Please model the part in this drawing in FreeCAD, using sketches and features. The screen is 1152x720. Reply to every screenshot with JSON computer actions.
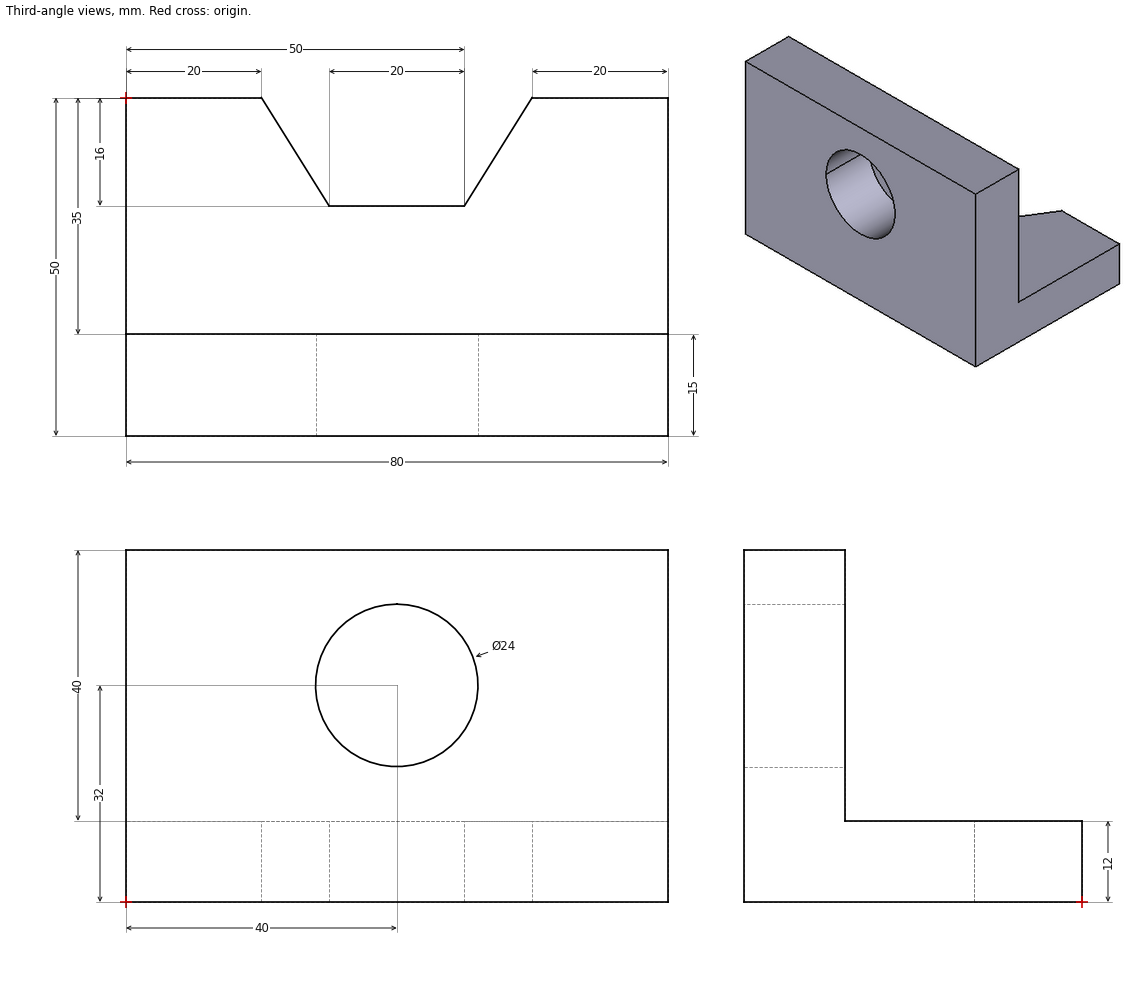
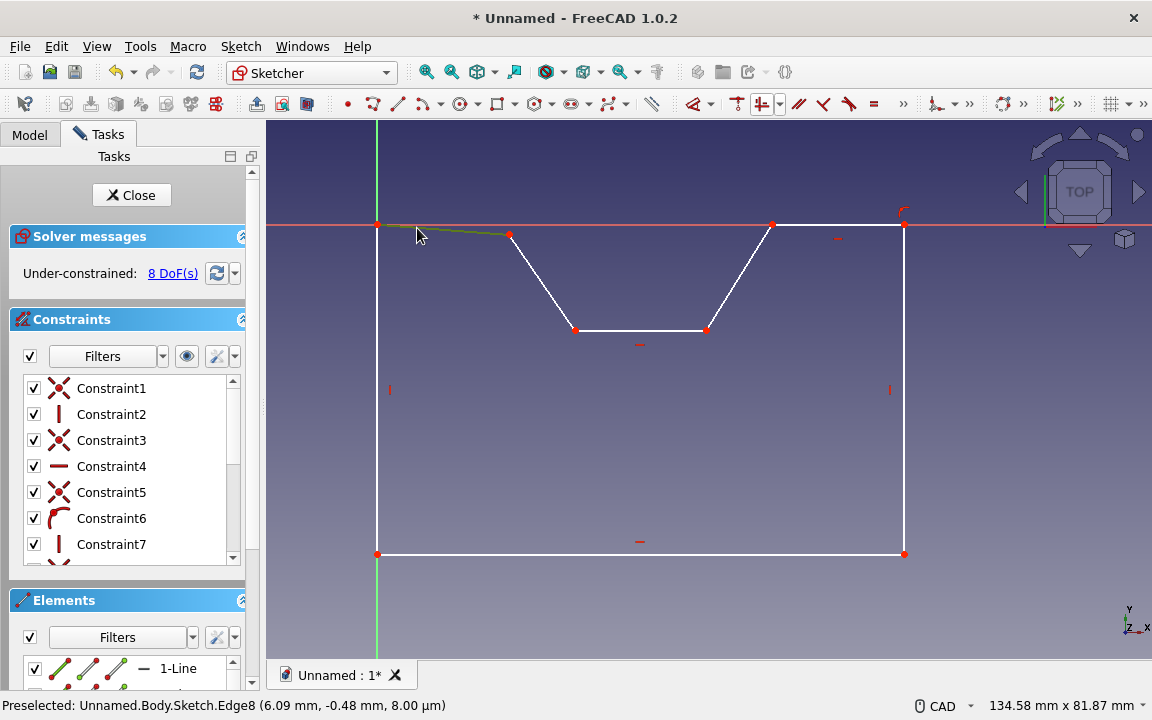
{"action": "left_click", "coordinate": [780, 104]}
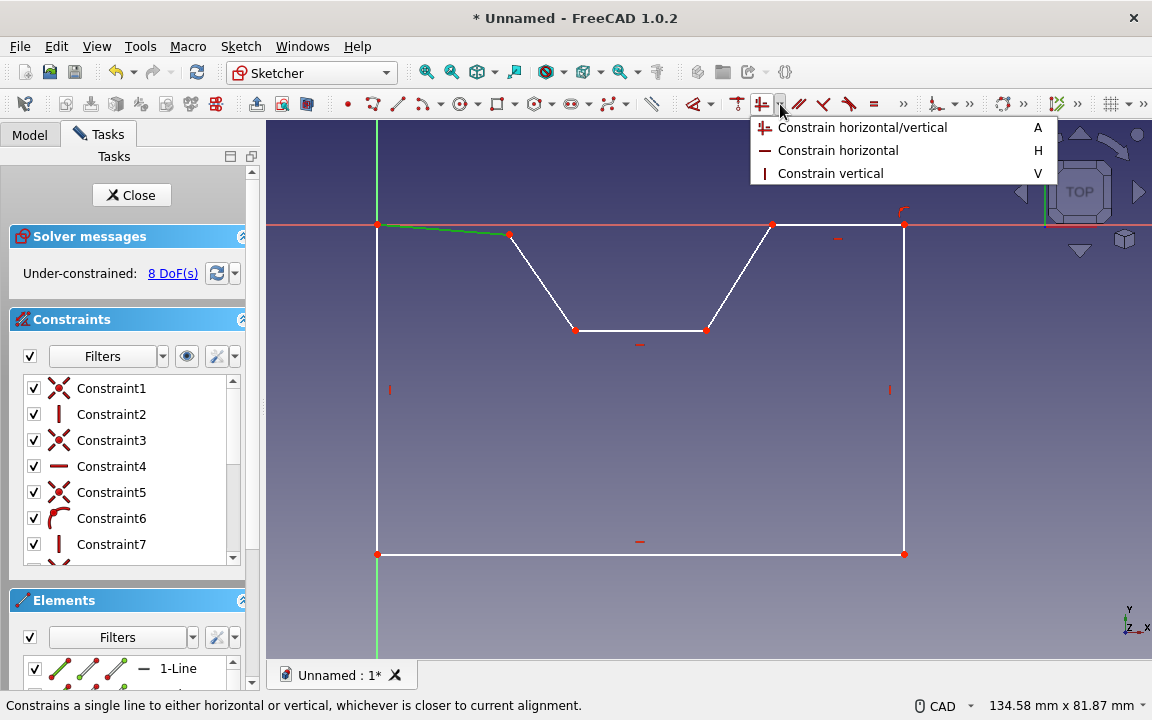
{"action": "left_click", "coordinate": [904, 150]}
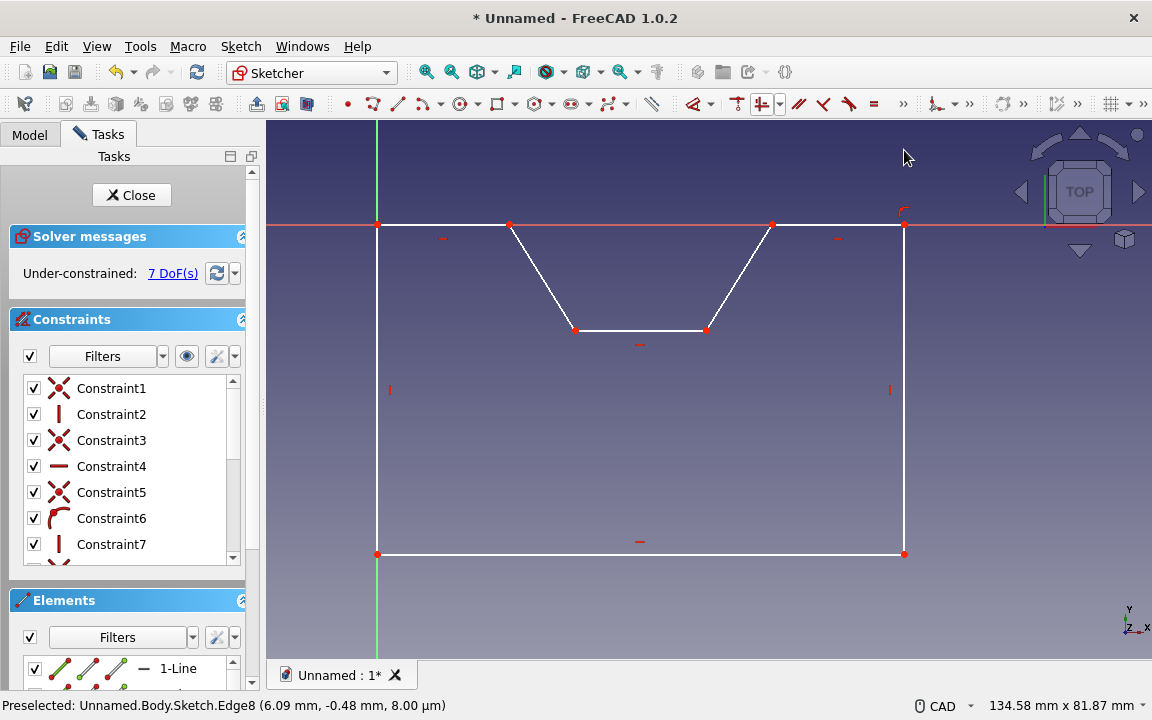
{"action": "left_click", "coordinate": [692, 104]}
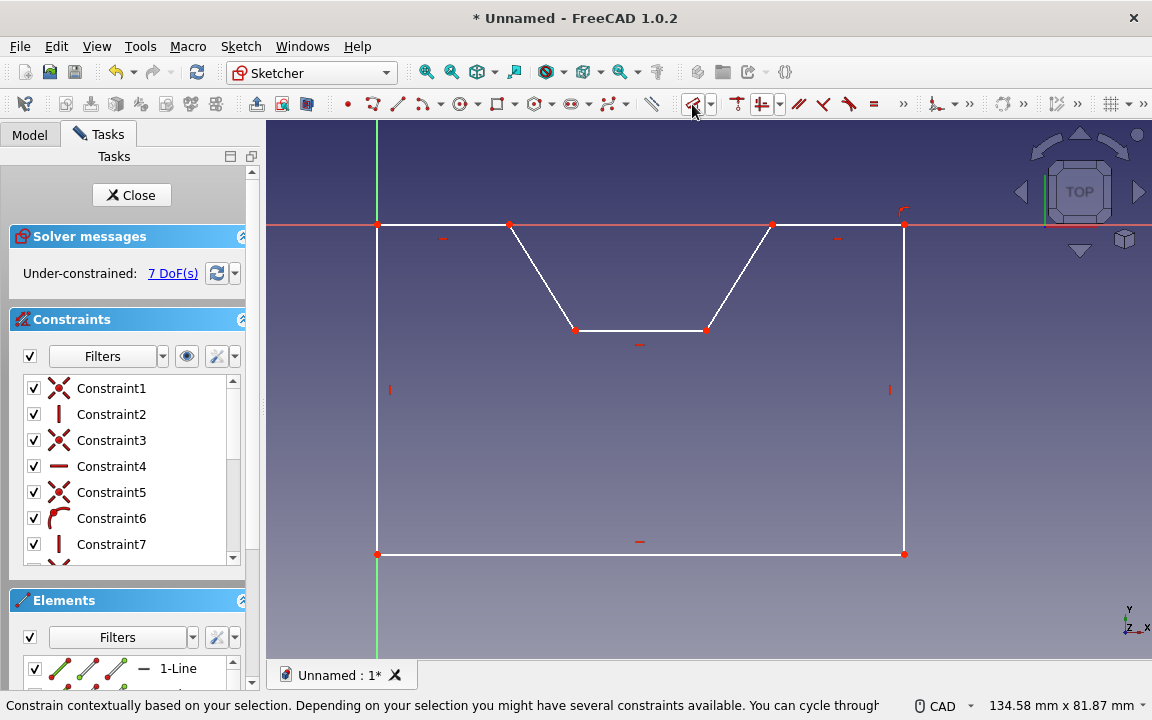
{"action": "left_click", "coordinate": [377, 324]}
{"action": "left_click", "coordinate": [343, 390]}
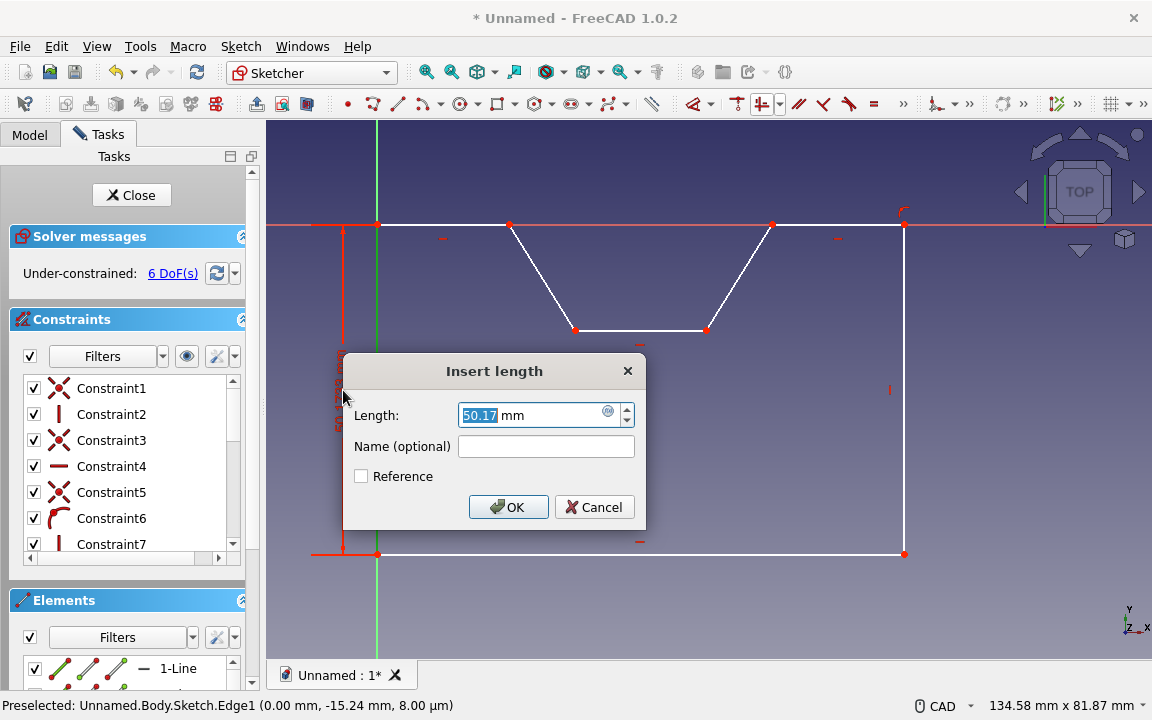
{"action": "type", "text": "50"}
{"action": "key", "text": "Return"}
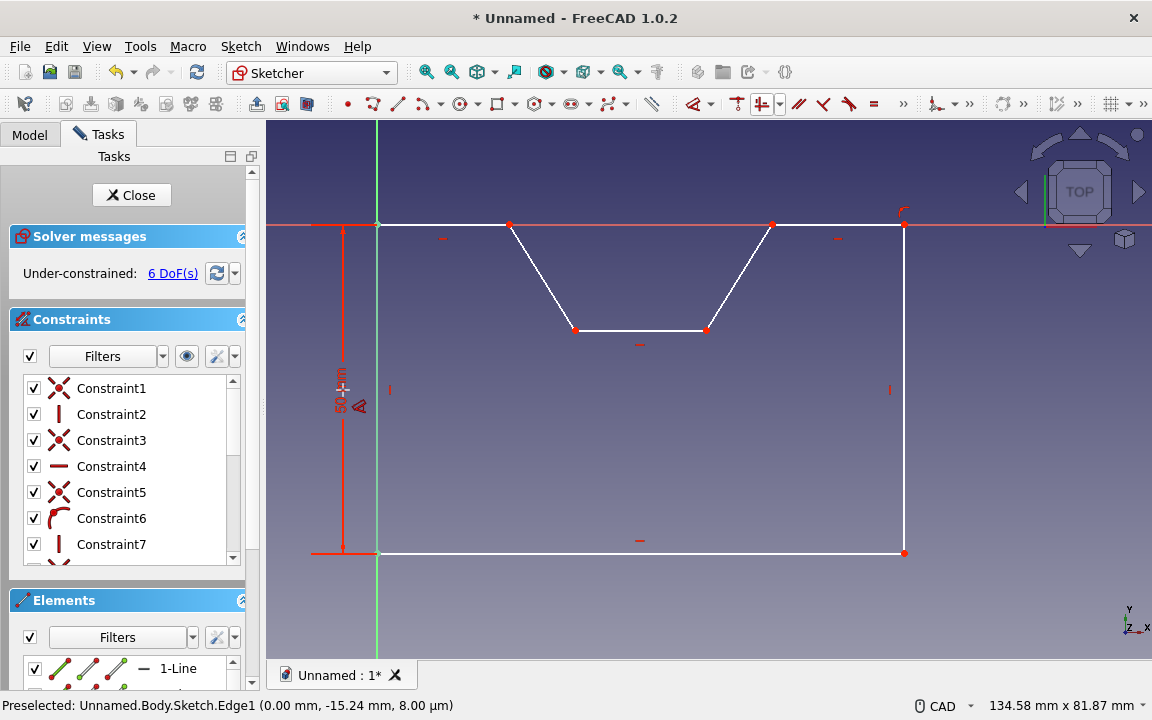
{"action": "left_click", "coordinate": [535, 554]}
{"action": "left_click", "coordinate": [641, 588]}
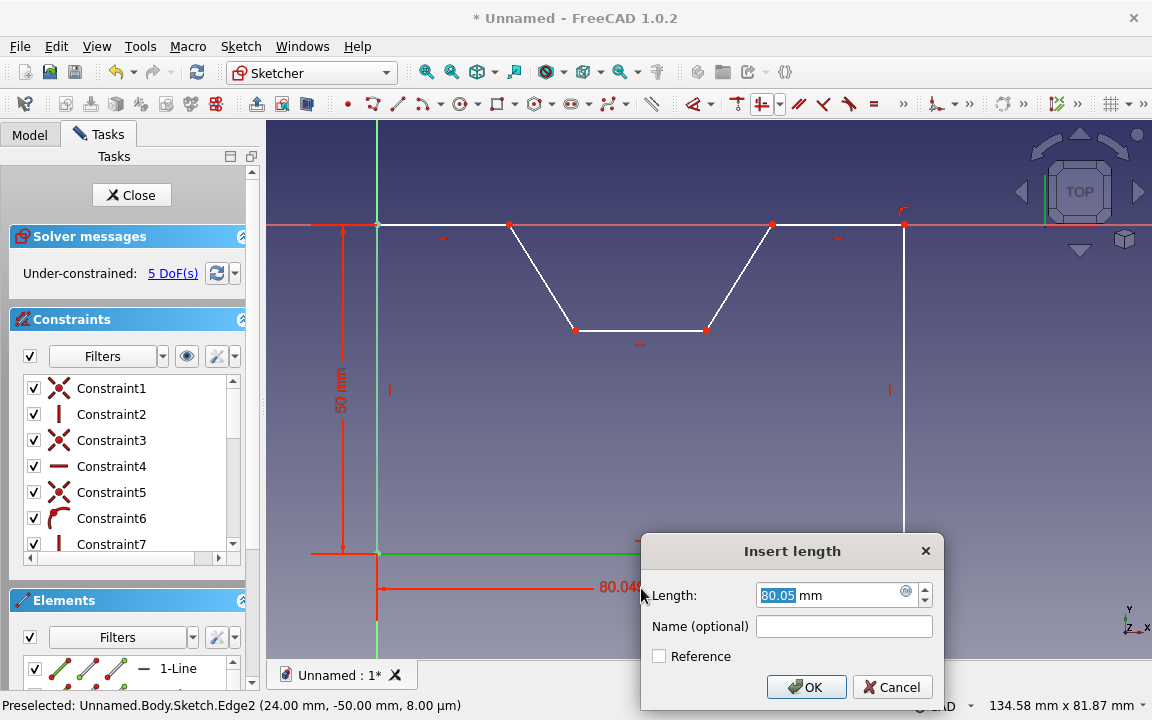
{"action": "type", "text": "80"}
{"action": "key", "text": "Return"}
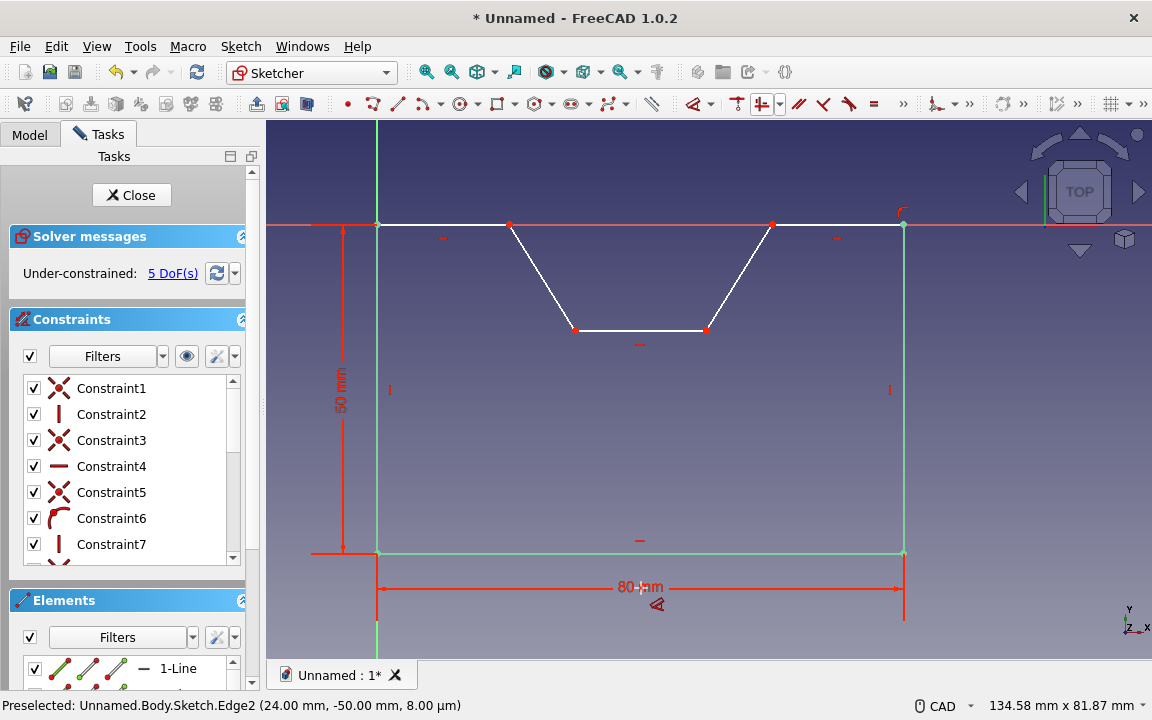
{"action": "left_click", "coordinate": [864, 225]}
{"action": "left_click", "coordinate": [838, 191]}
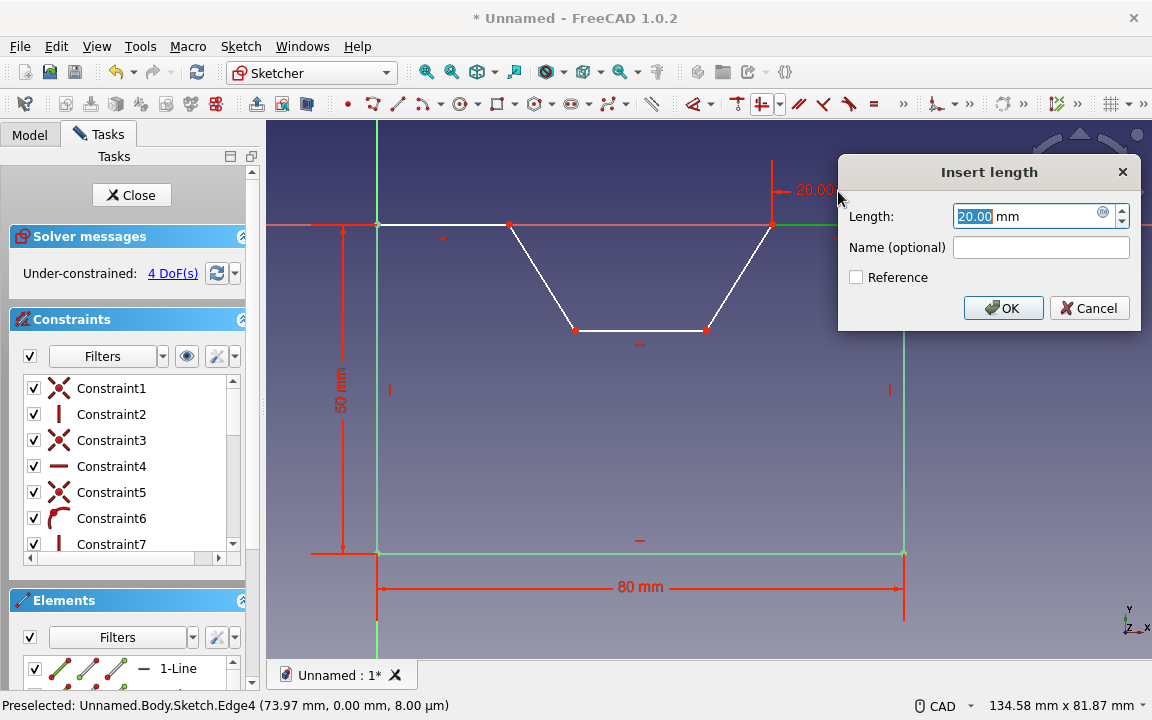
{"action": "type", "text": "20"}
{"action": "key", "text": "Return"}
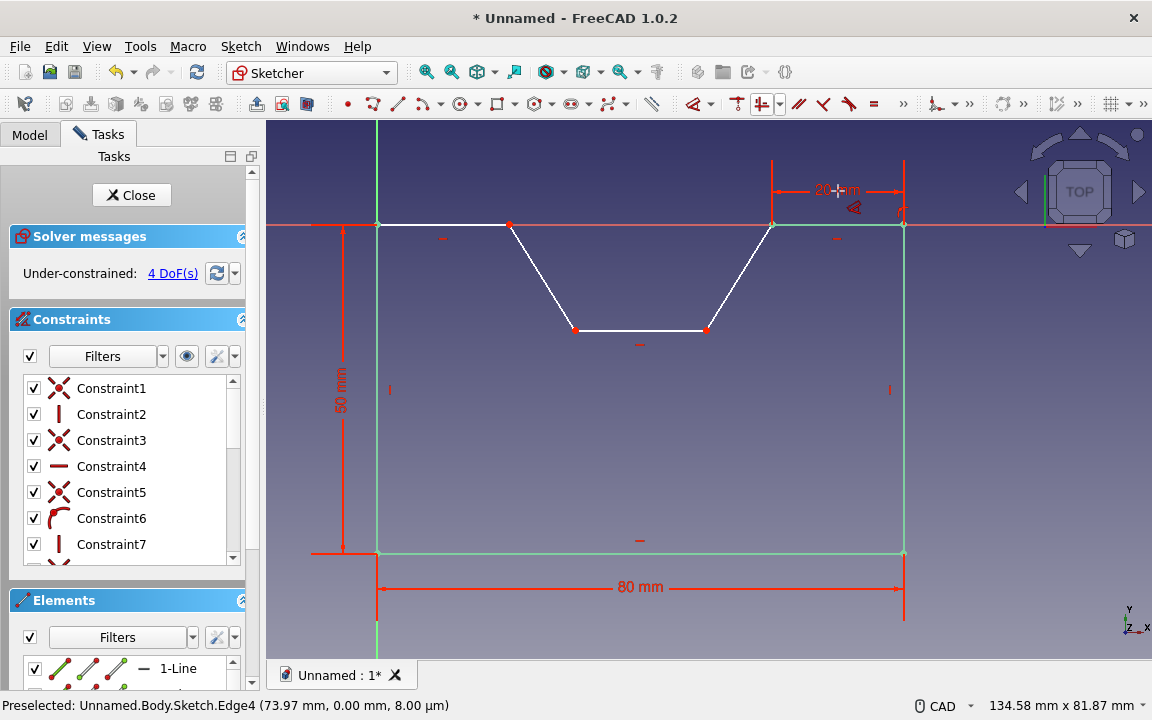
{"action": "left_click", "coordinate": [667, 331]}
{"action": "left_click", "coordinate": [641, 297]}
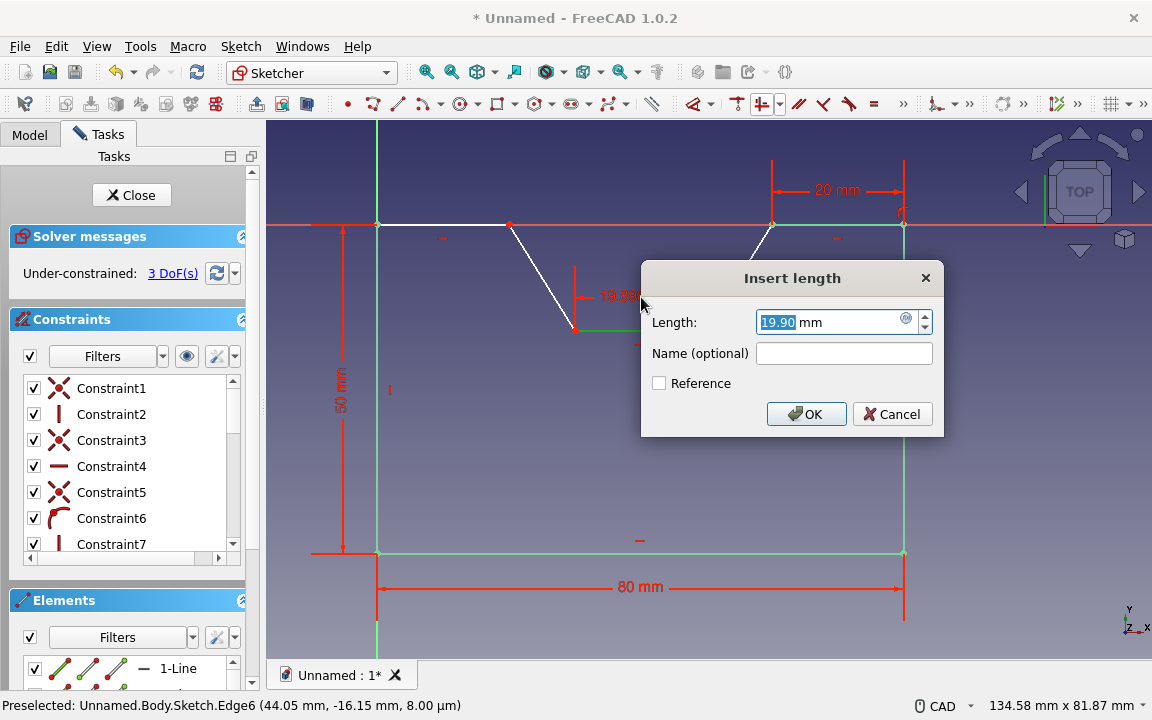
{"action": "type", "text": "20"}
{"action": "key", "text": "Return"}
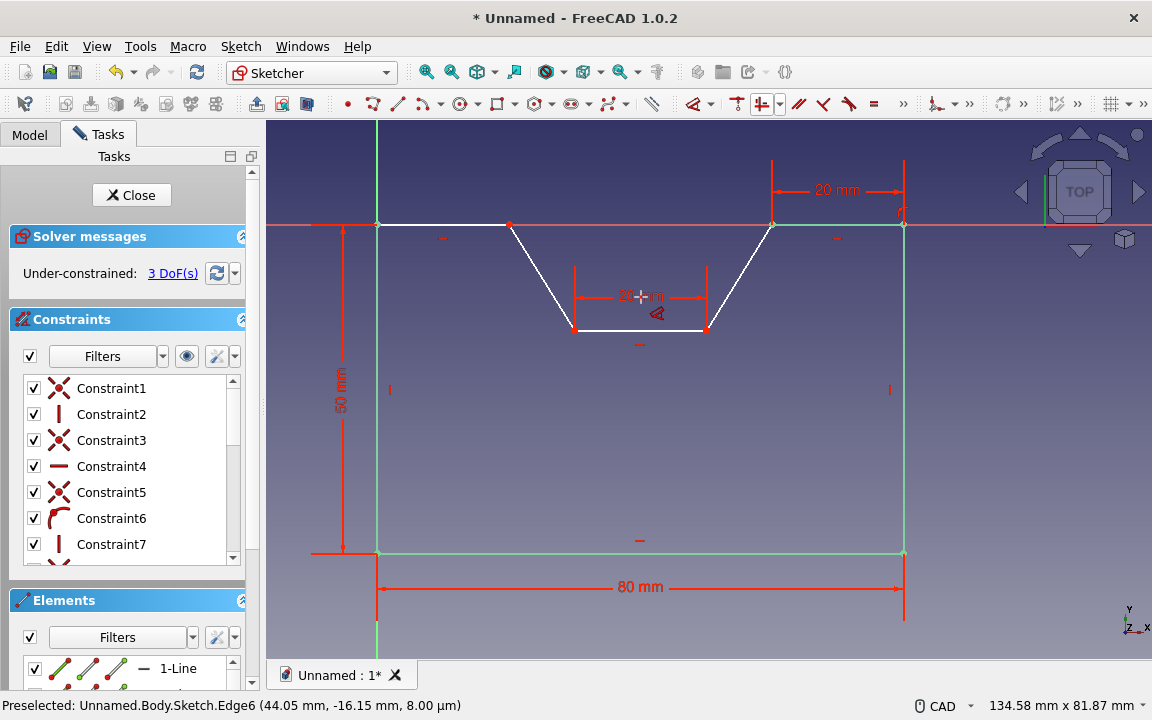
{"action": "left_click", "coordinate": [469, 225]}
{"action": "left_click", "coordinate": [443, 191]}